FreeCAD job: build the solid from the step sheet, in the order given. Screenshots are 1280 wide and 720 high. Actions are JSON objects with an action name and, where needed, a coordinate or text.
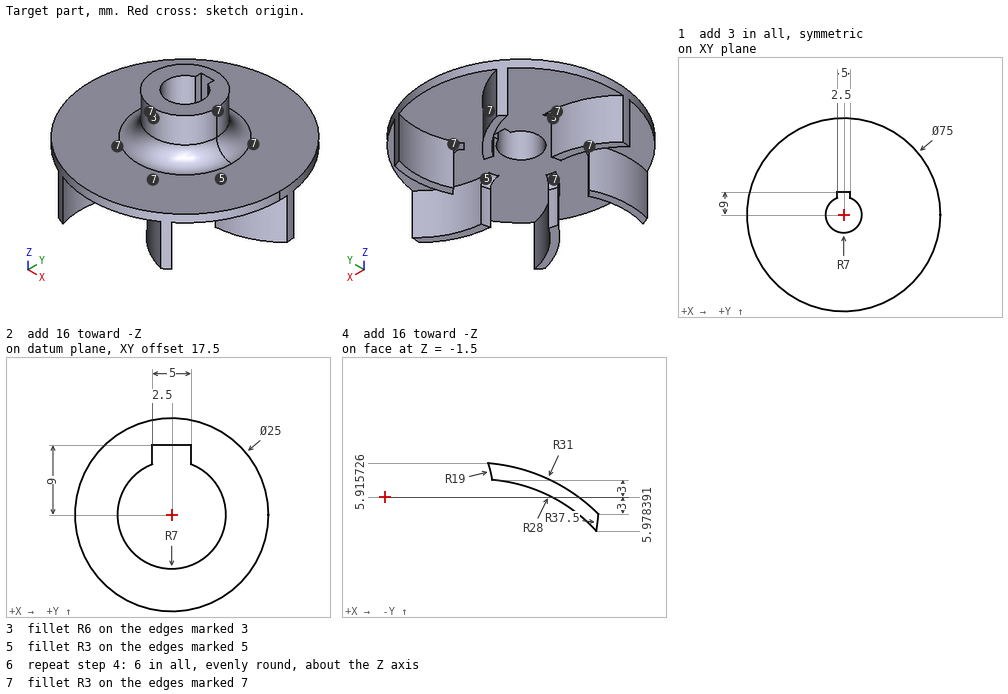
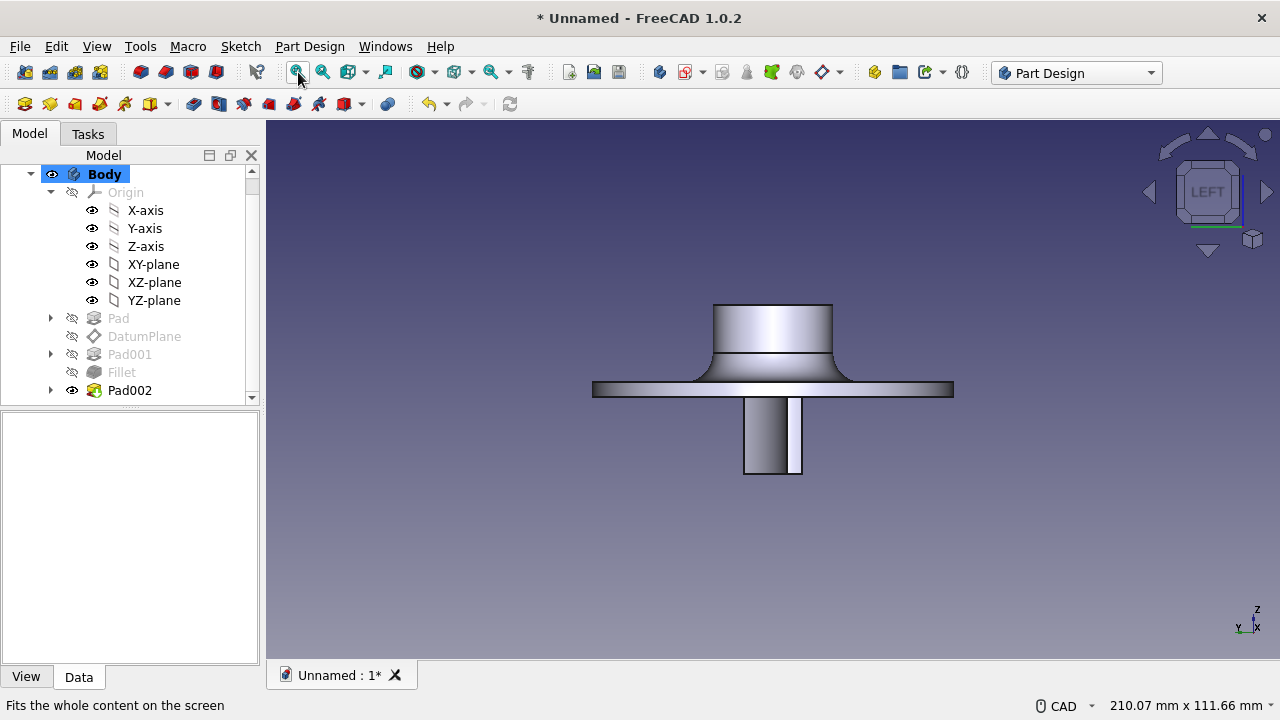
{"action": "key", "text": "v 3"}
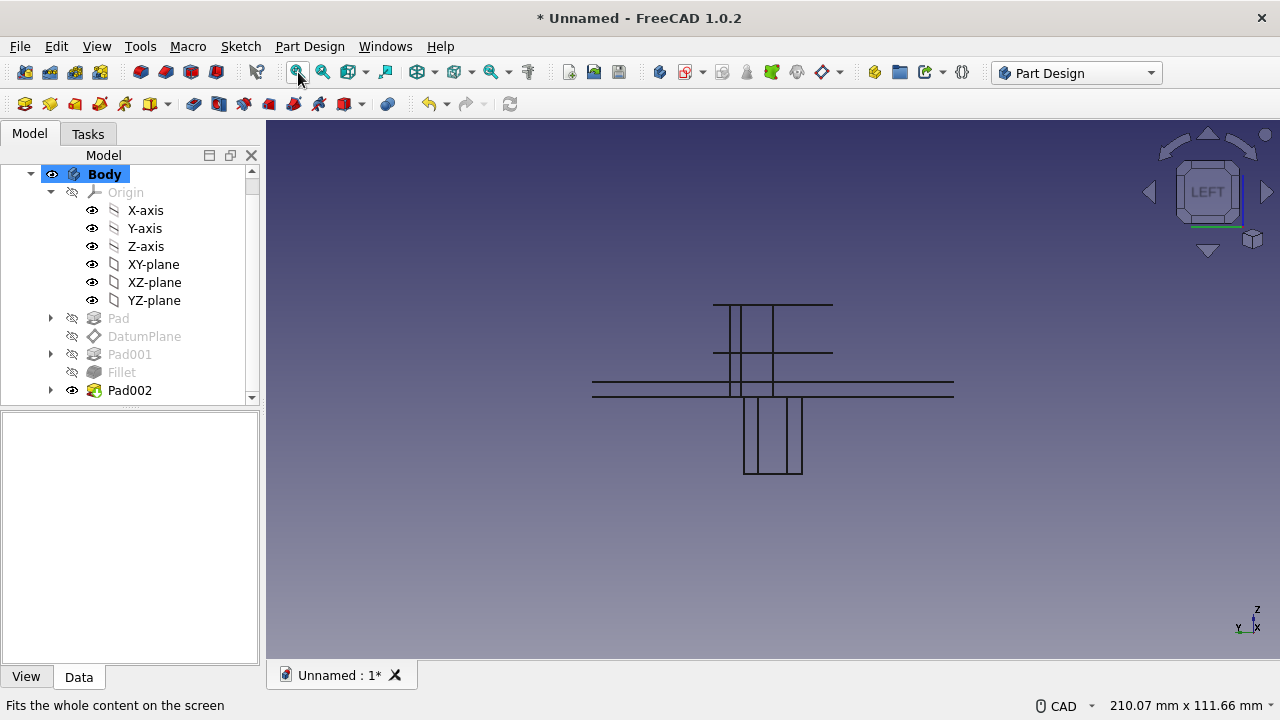
{"action": "key", "text": "0"}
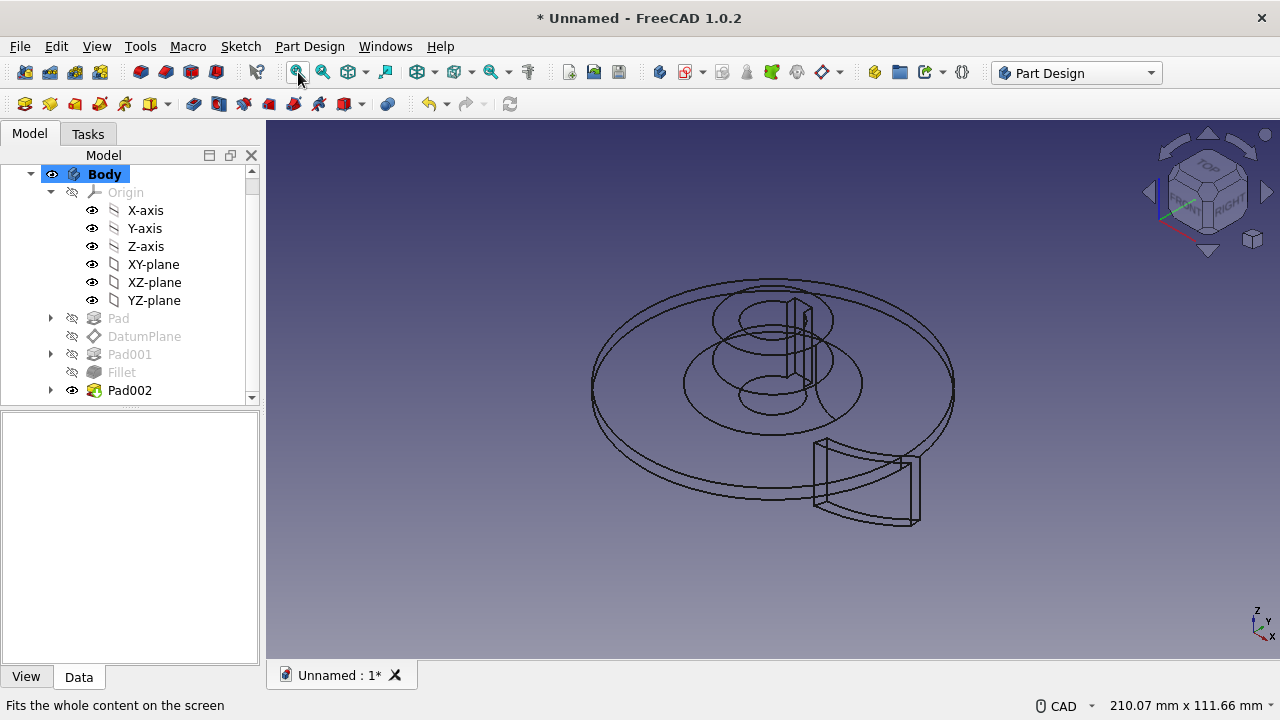
{"action": "left_click", "coordinate": [824, 438]}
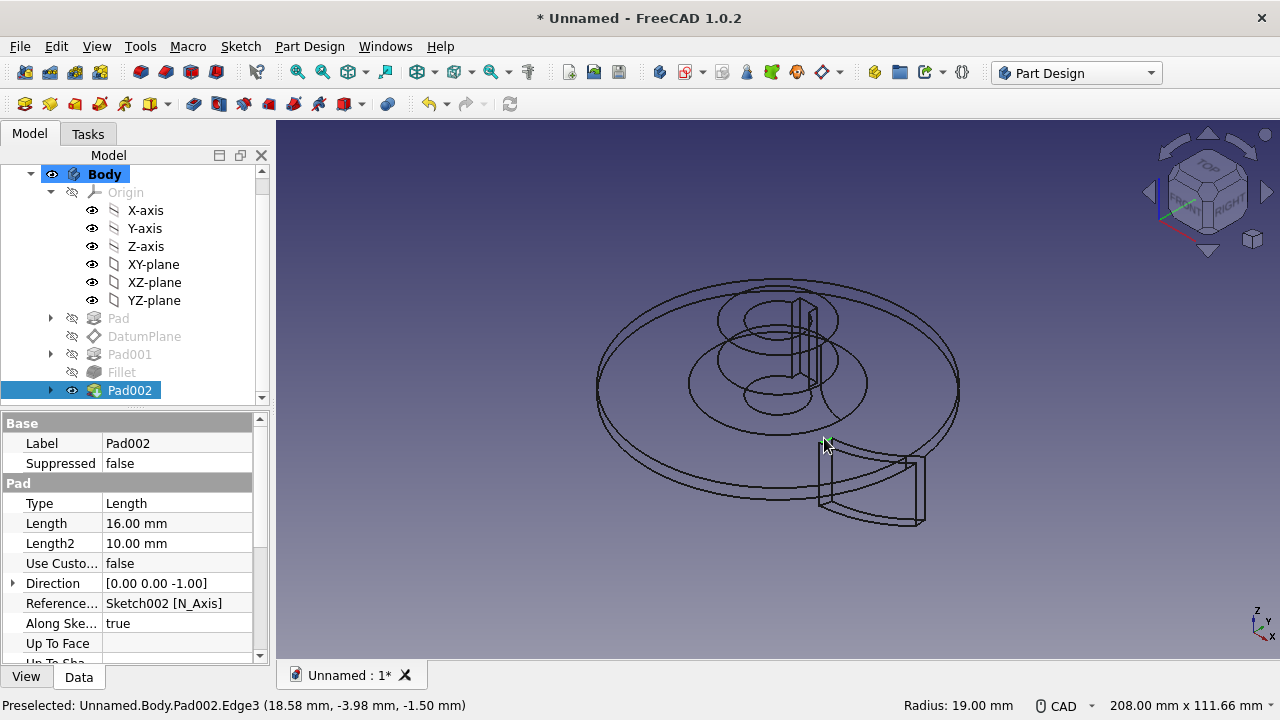
{"action": "key", "text": "v 1"}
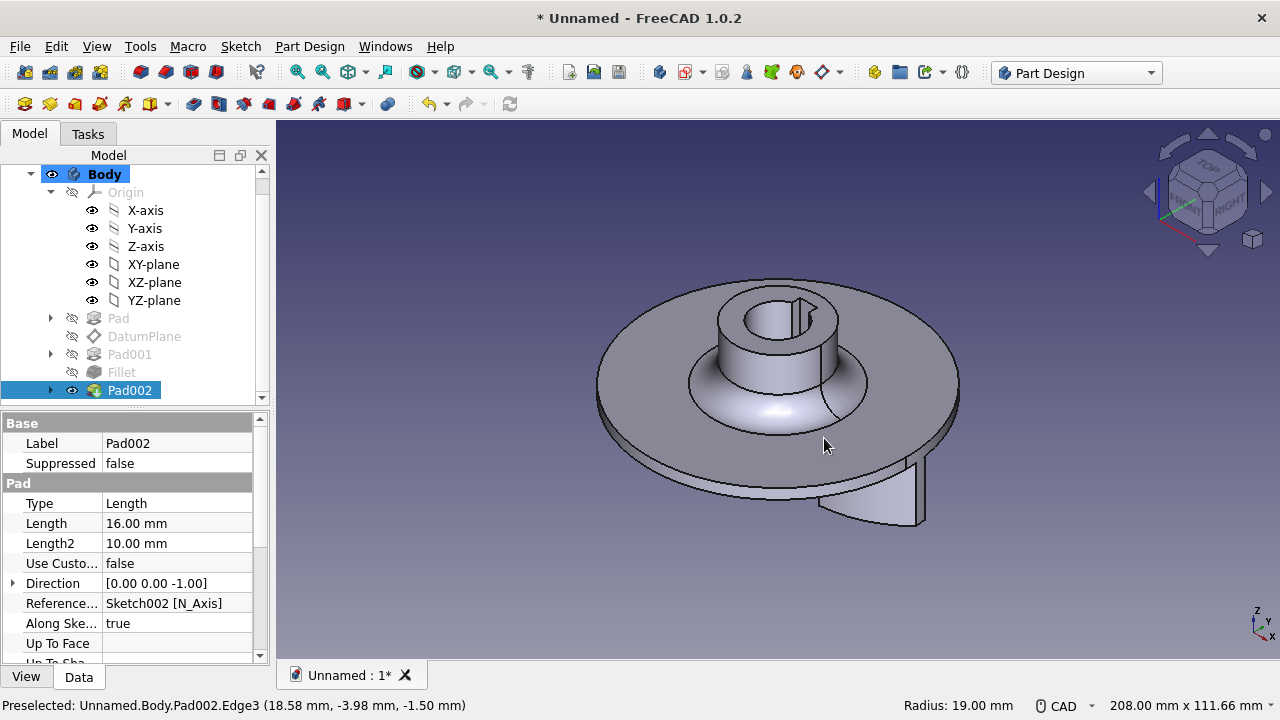
{"action": "left_click", "coordinate": [141, 72]}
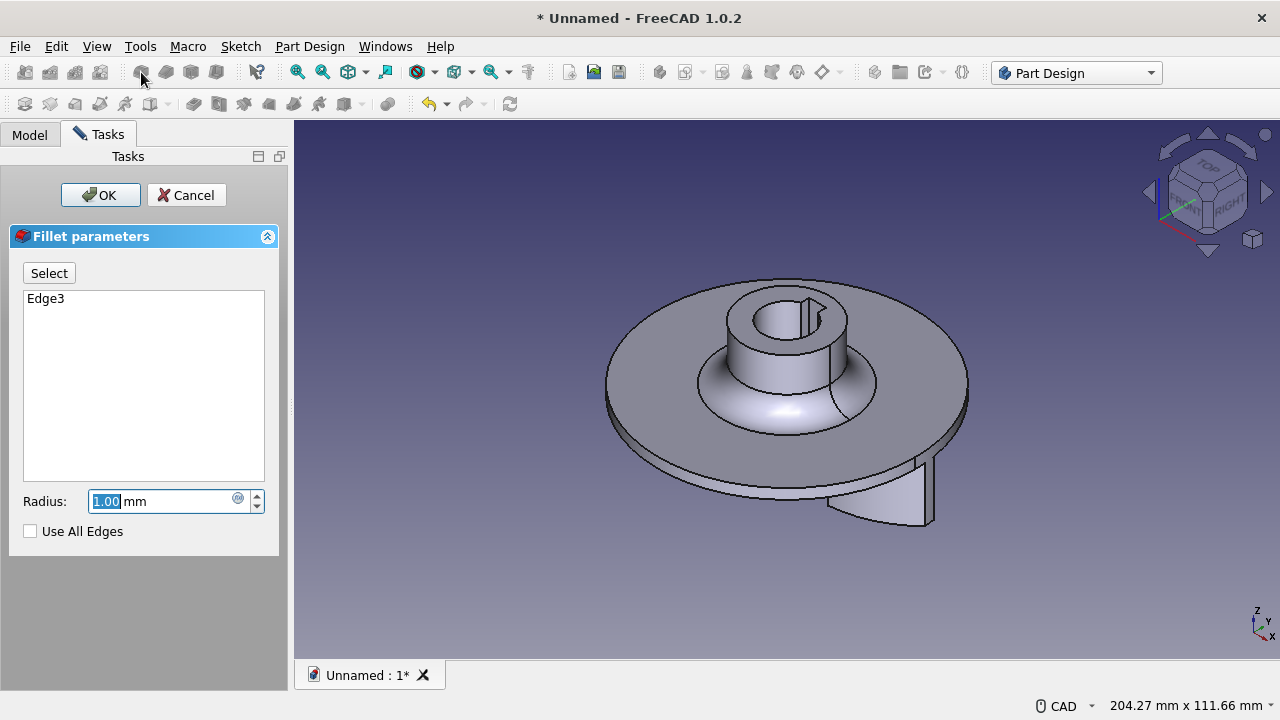
{"action": "type", "text": "3"}
{"action": "key", "text": "Tab"}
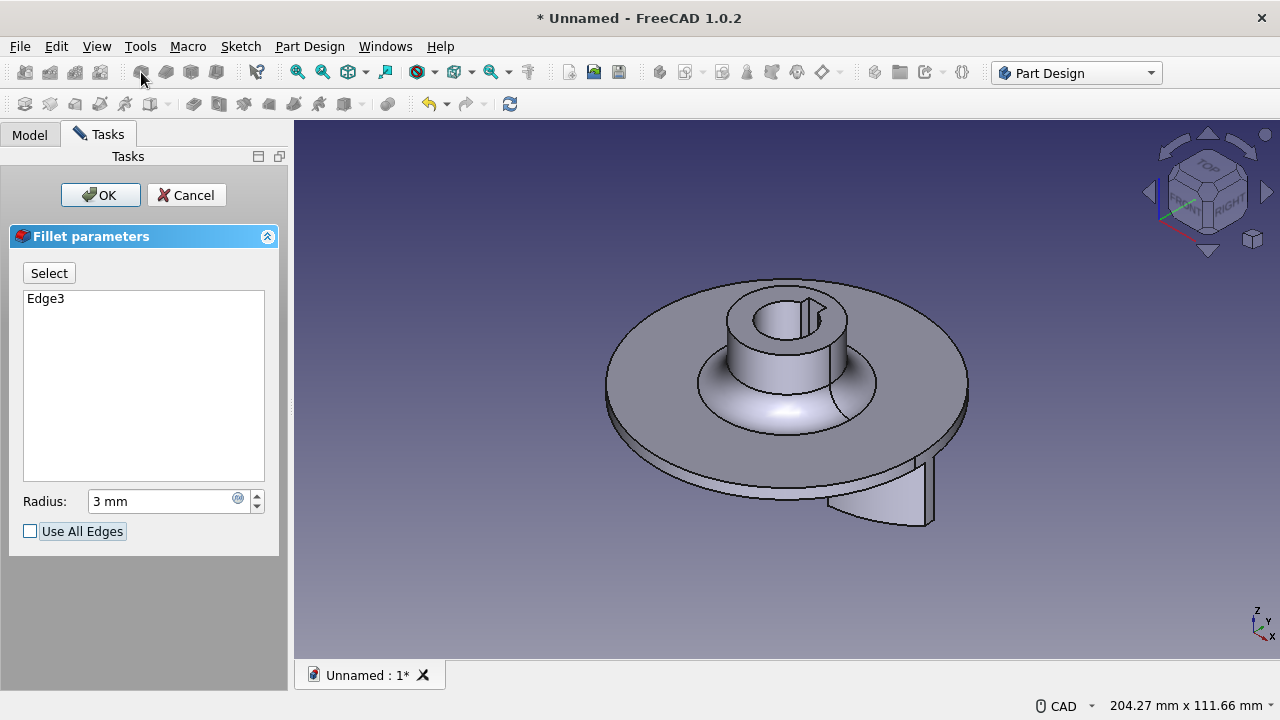
{"action": "left_click", "coordinate": [101, 195]}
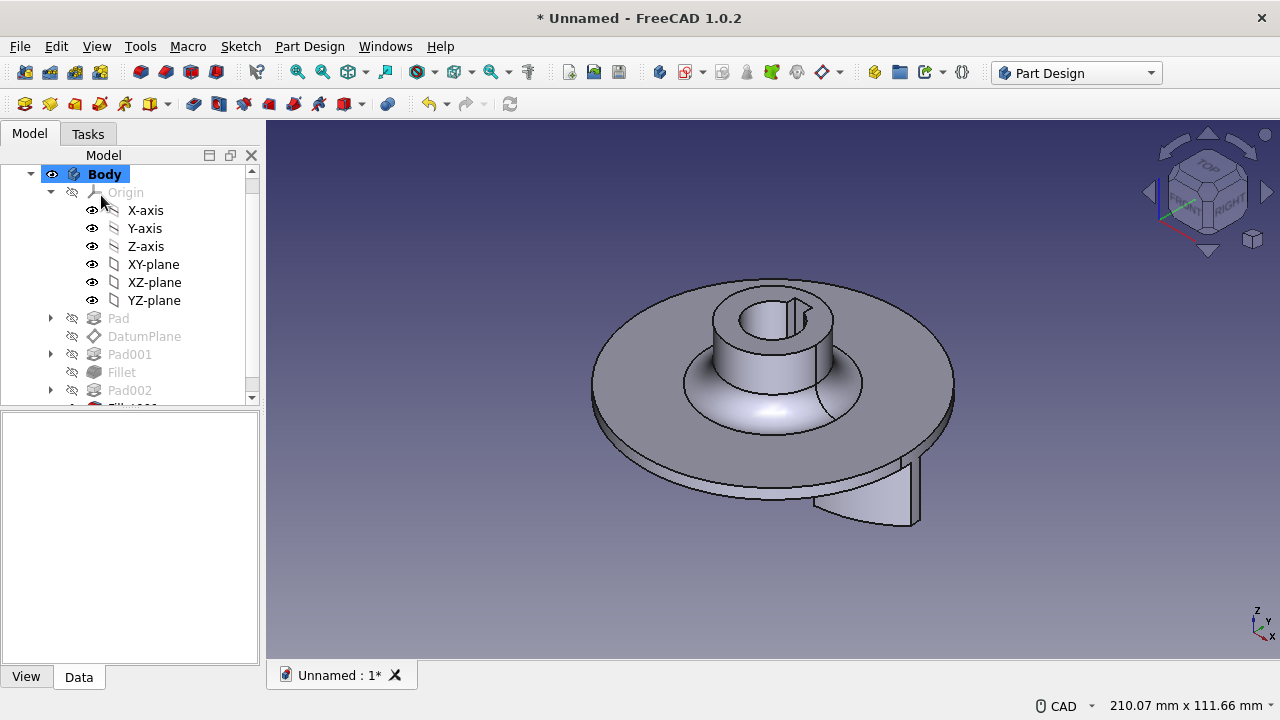
{"action": "left_click", "coordinate": [117, 390]}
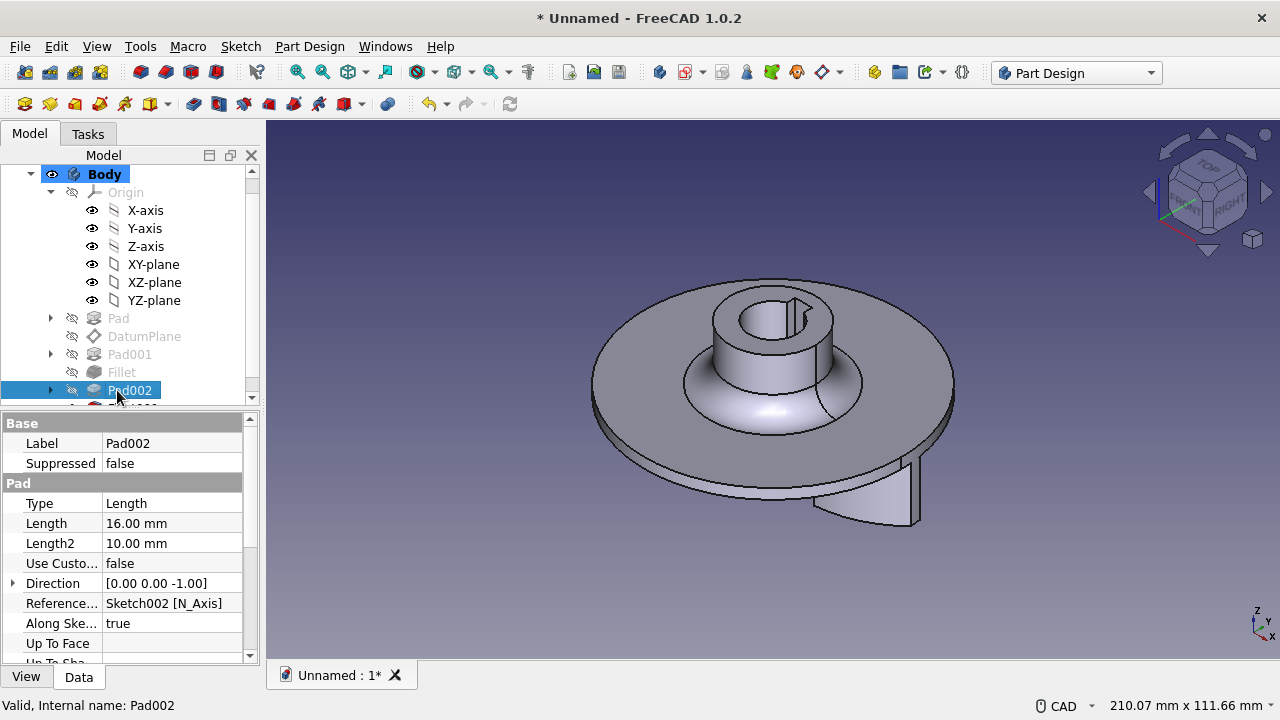
{"action": "left_click", "coordinate": [75, 72]}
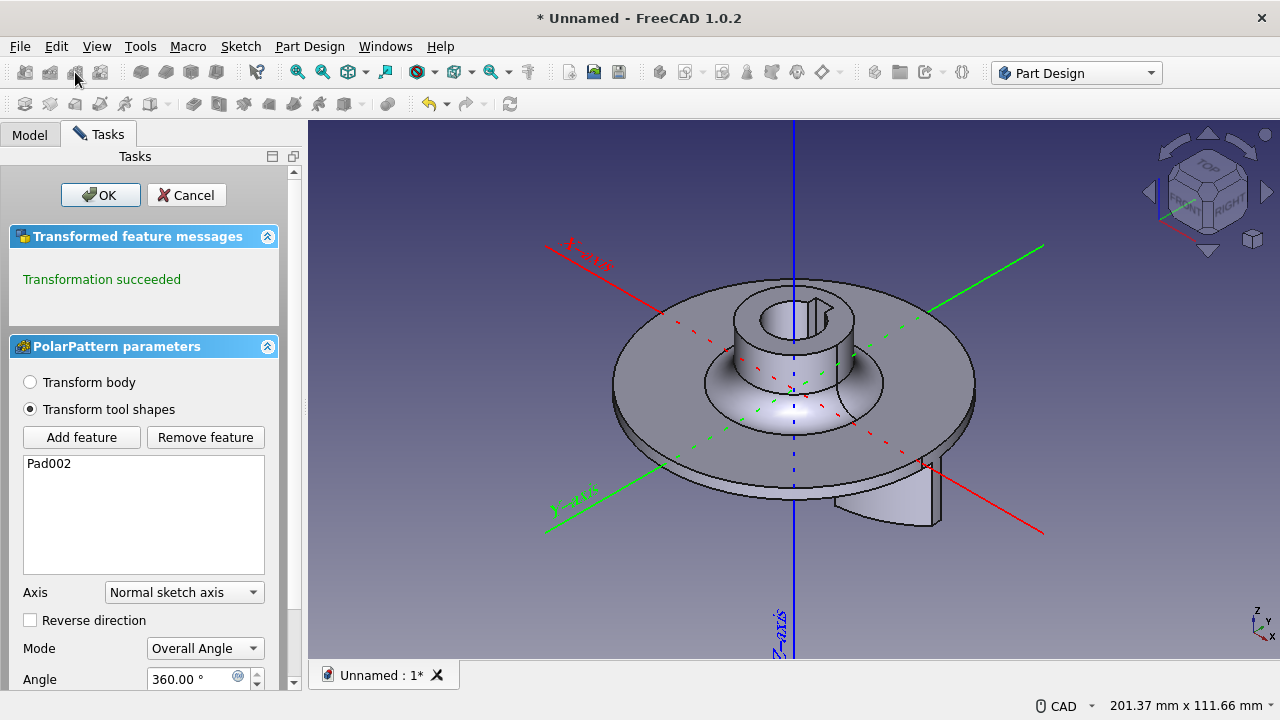
{"action": "left_click", "coordinate": [185, 592]}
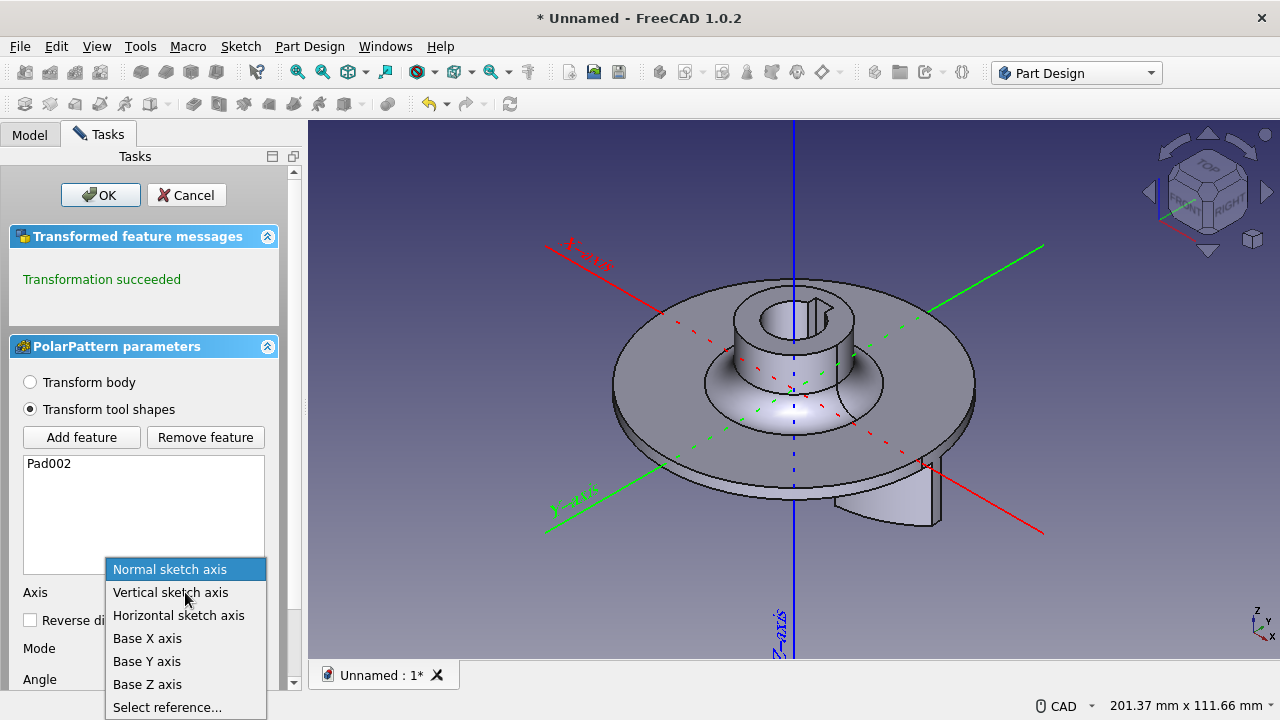
{"action": "left_click", "coordinate": [184, 684]}